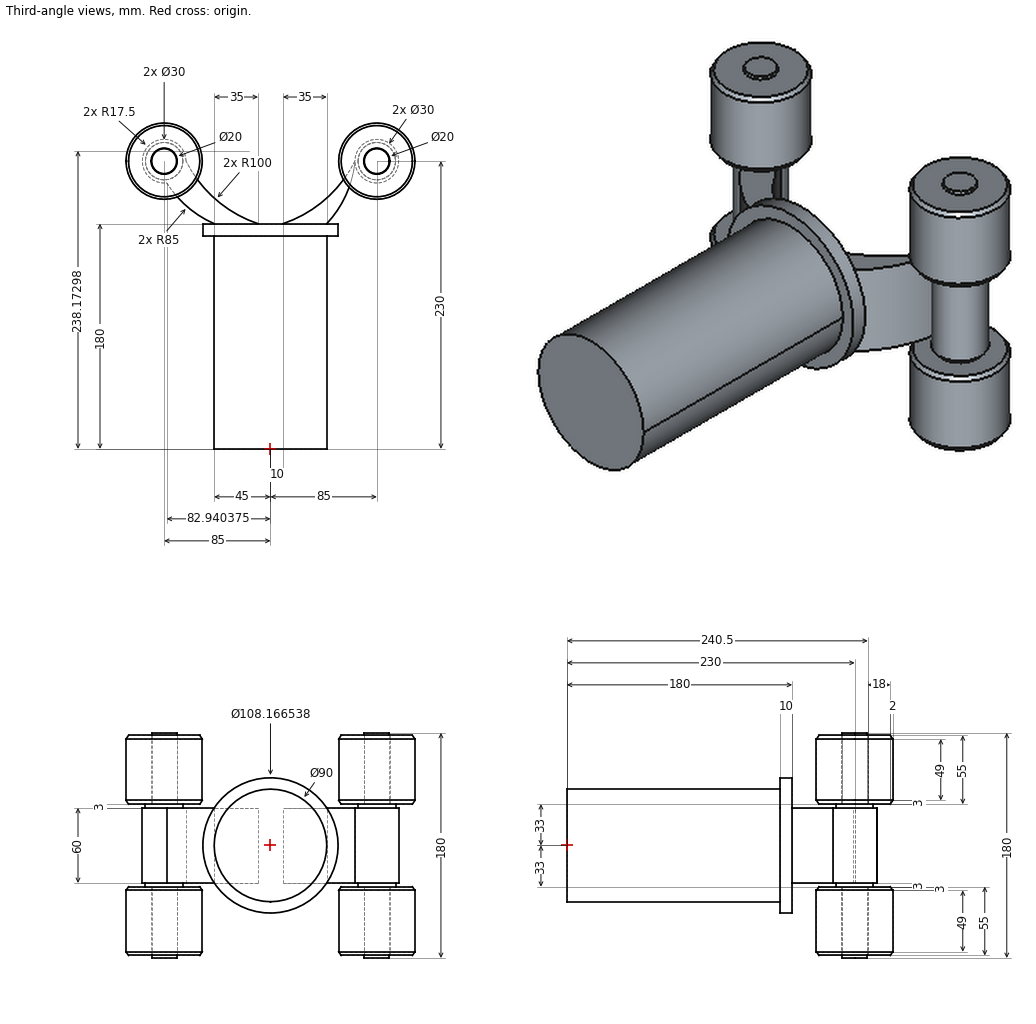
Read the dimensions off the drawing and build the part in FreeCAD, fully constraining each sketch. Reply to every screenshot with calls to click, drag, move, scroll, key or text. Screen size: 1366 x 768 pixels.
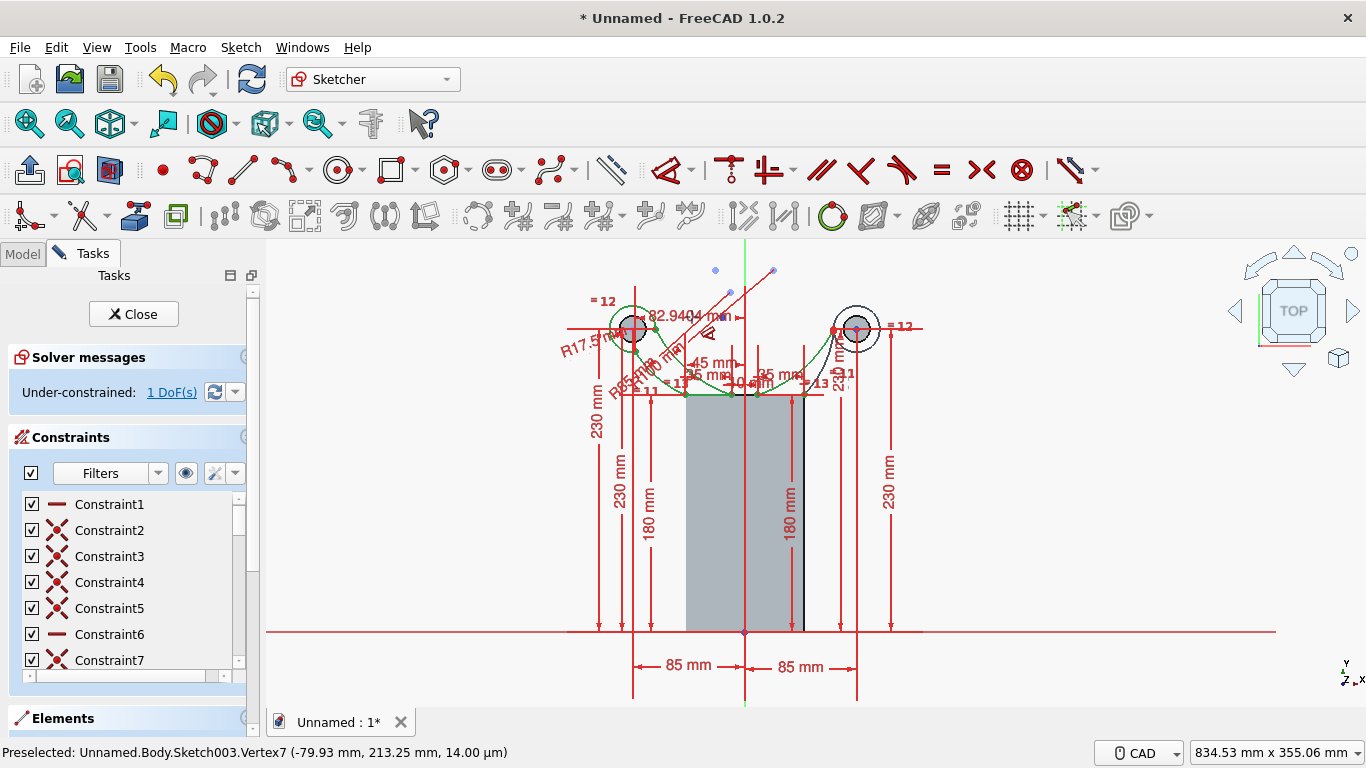
click(723, 318)
click(689, 547)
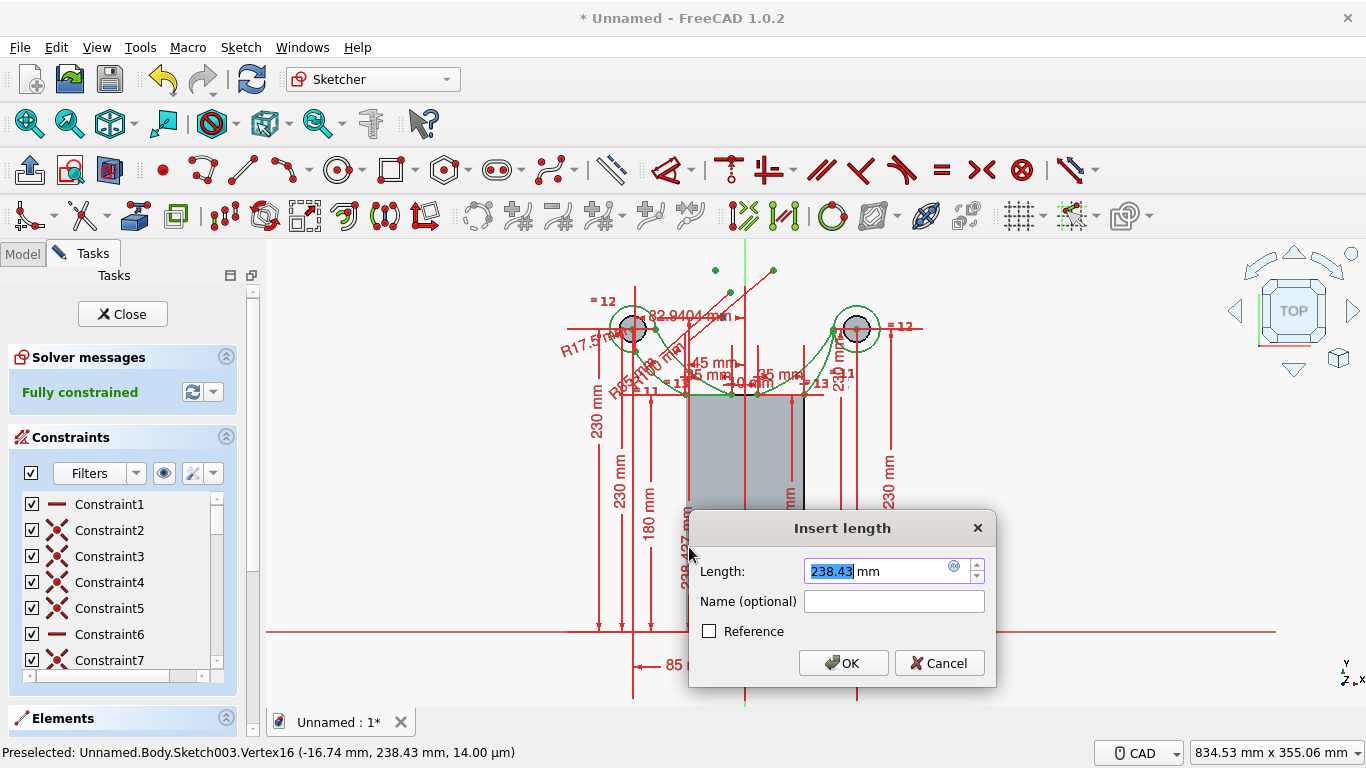
text(238.17298)
key(Return)
key(Escape)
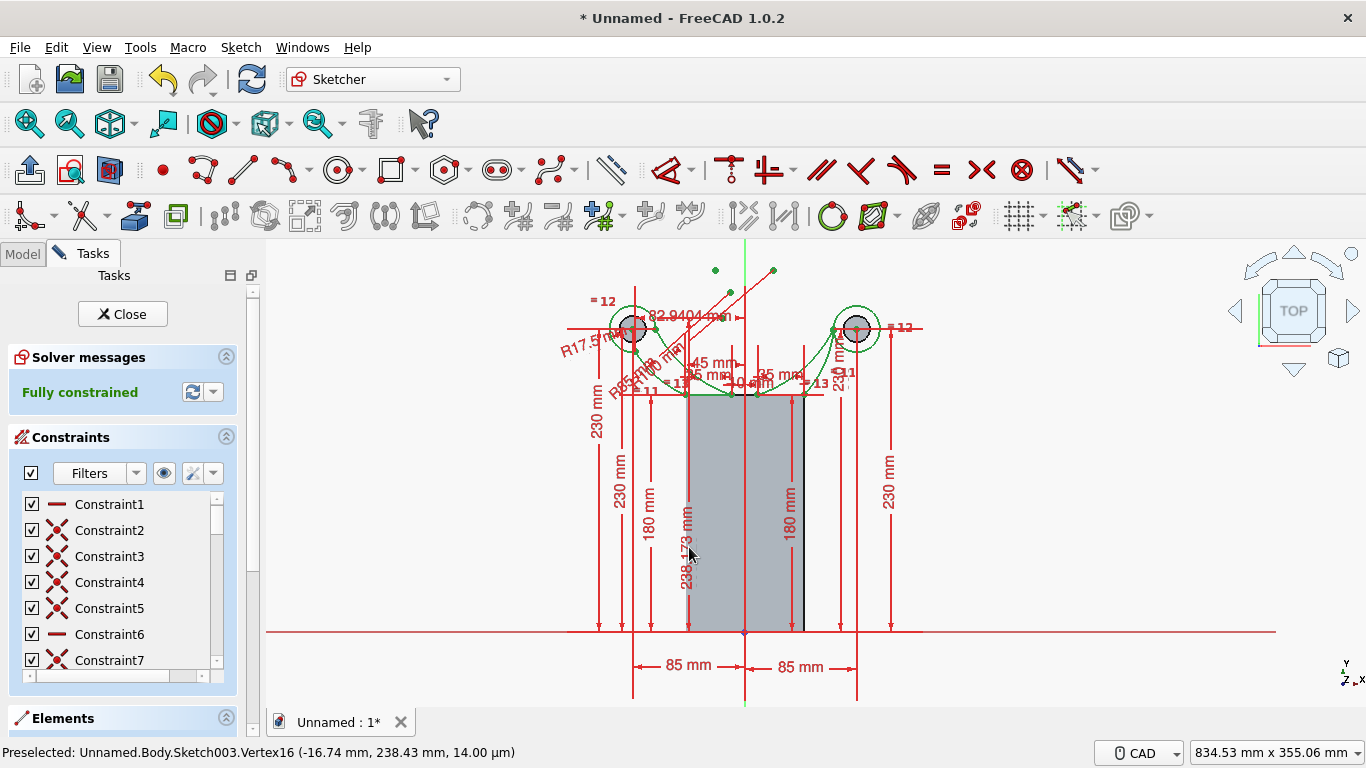
click(123, 314)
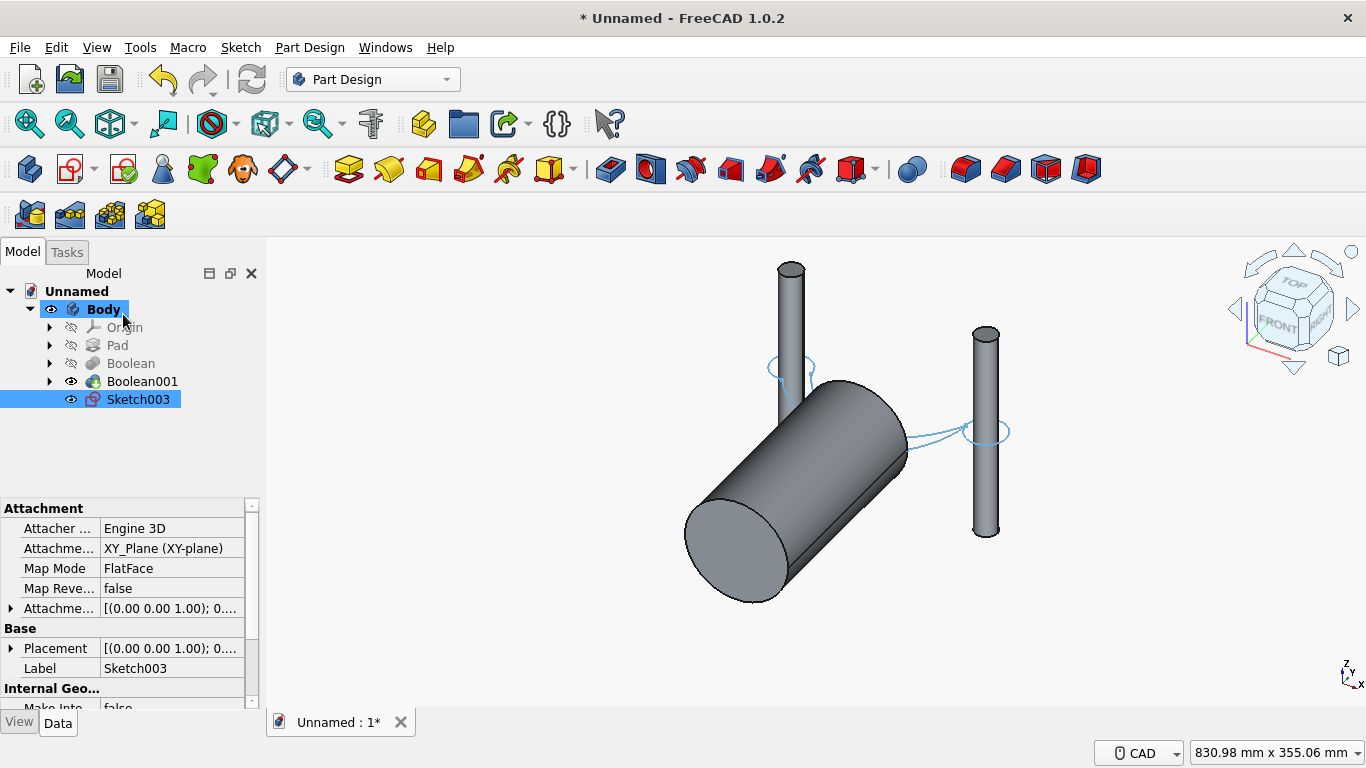
click(350, 170)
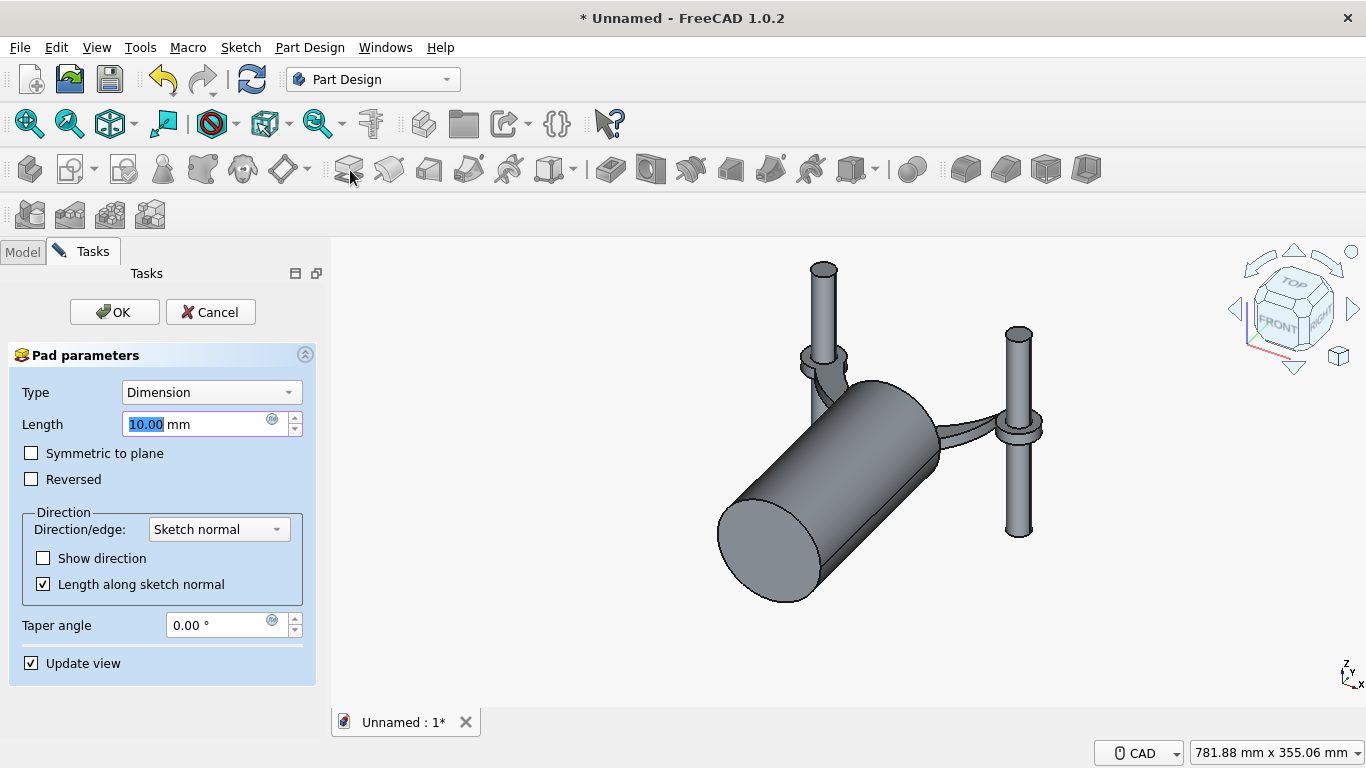
text(60)
key(Tab)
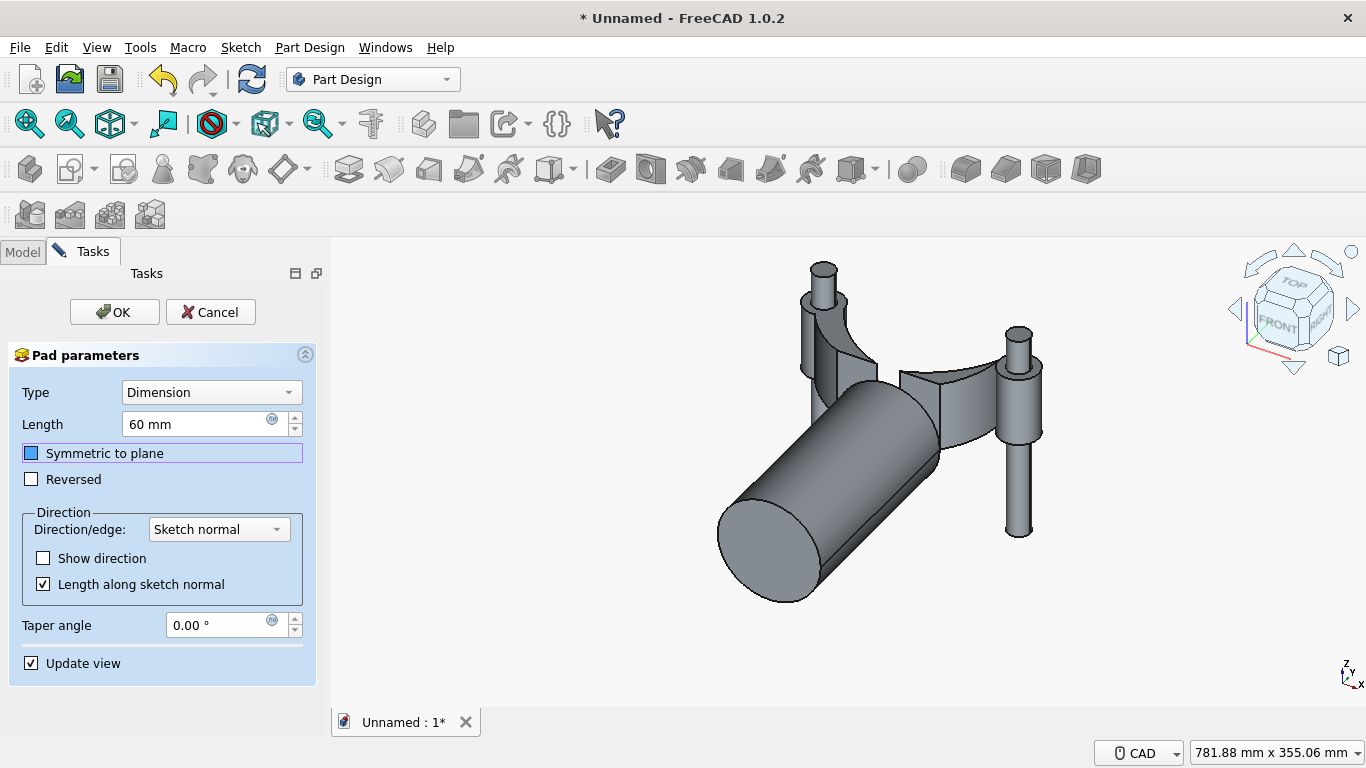
click(30, 453)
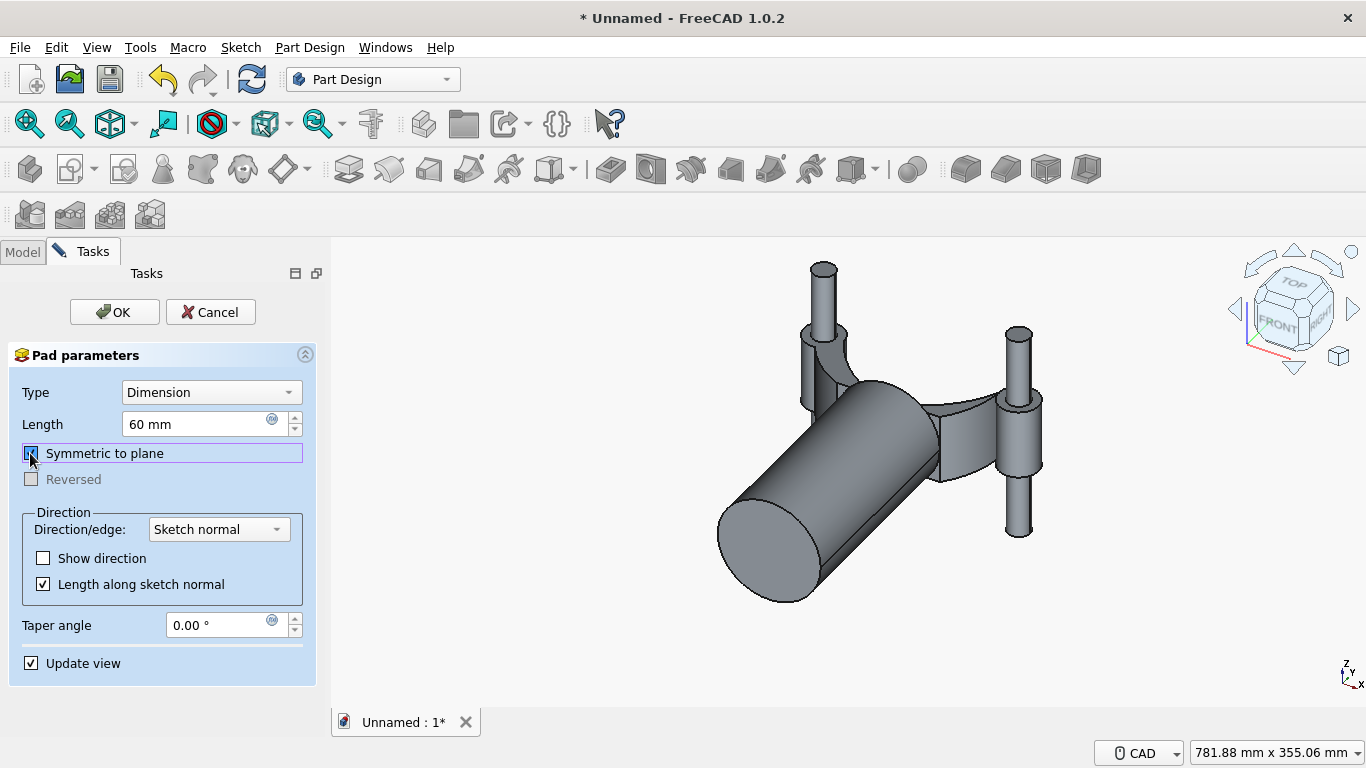
click(115, 312)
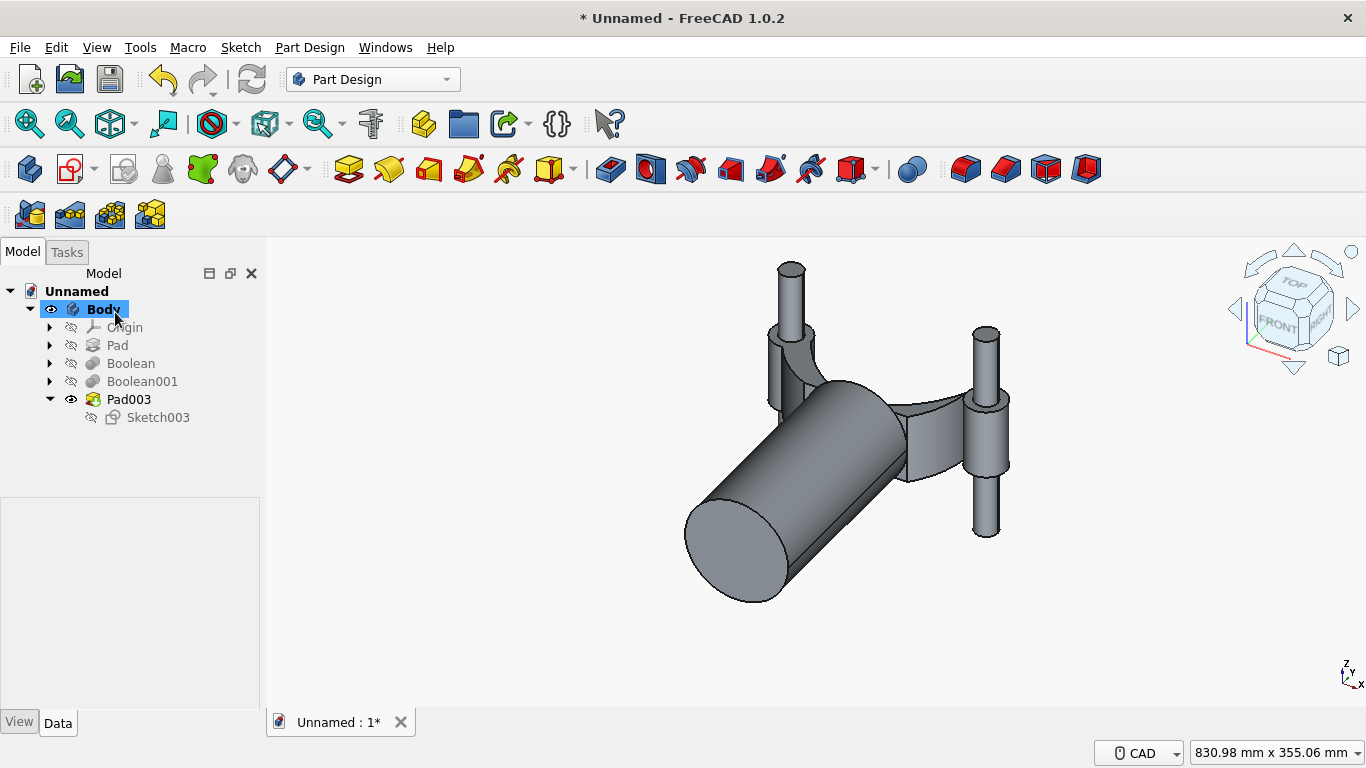
key(4)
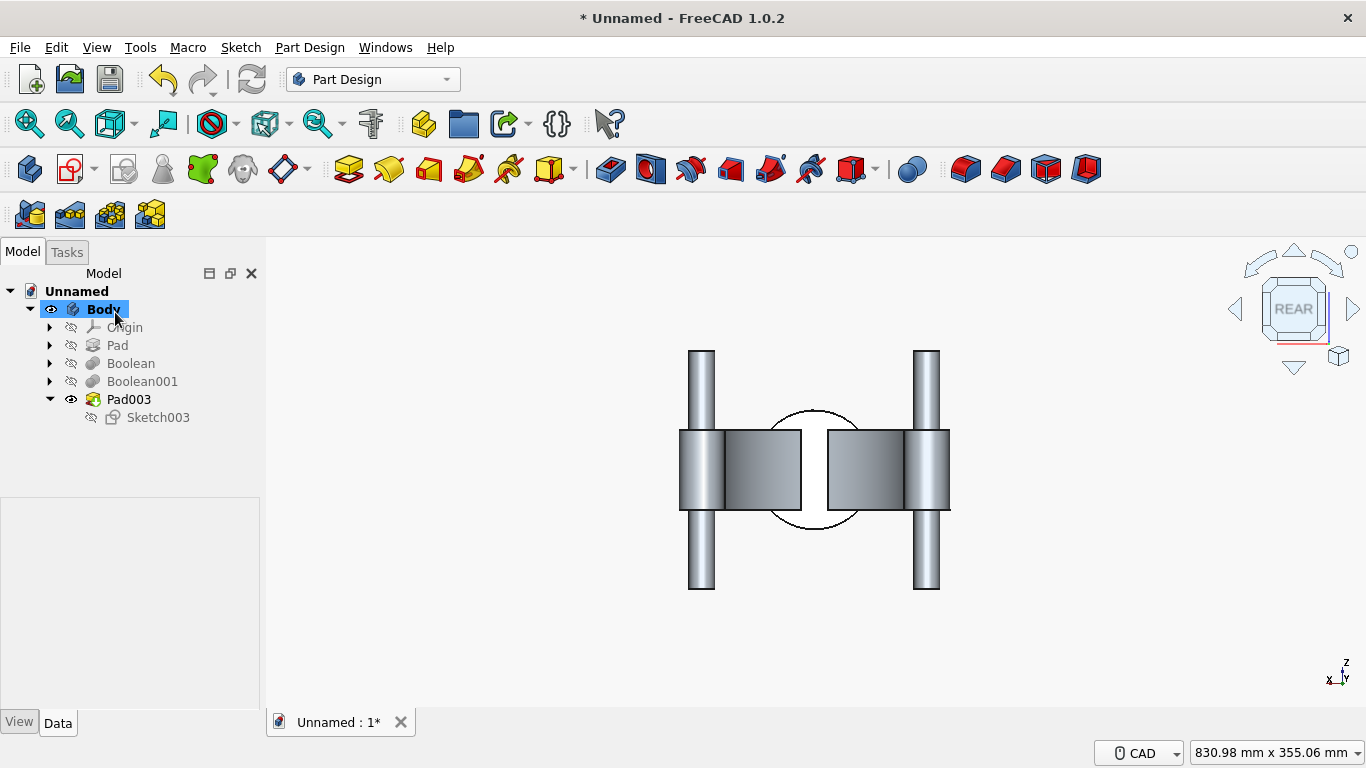
click(815, 435)